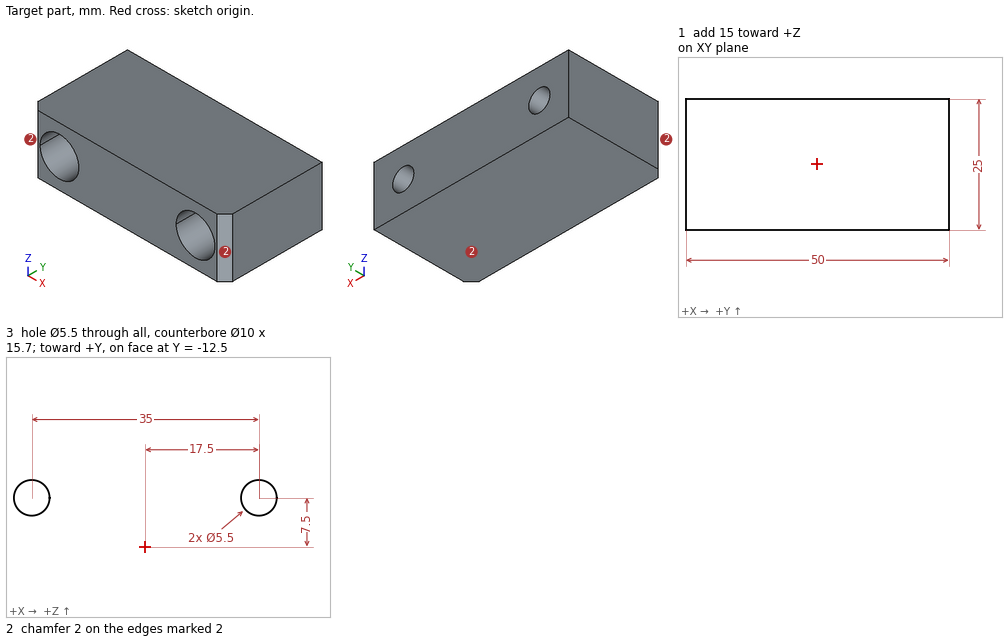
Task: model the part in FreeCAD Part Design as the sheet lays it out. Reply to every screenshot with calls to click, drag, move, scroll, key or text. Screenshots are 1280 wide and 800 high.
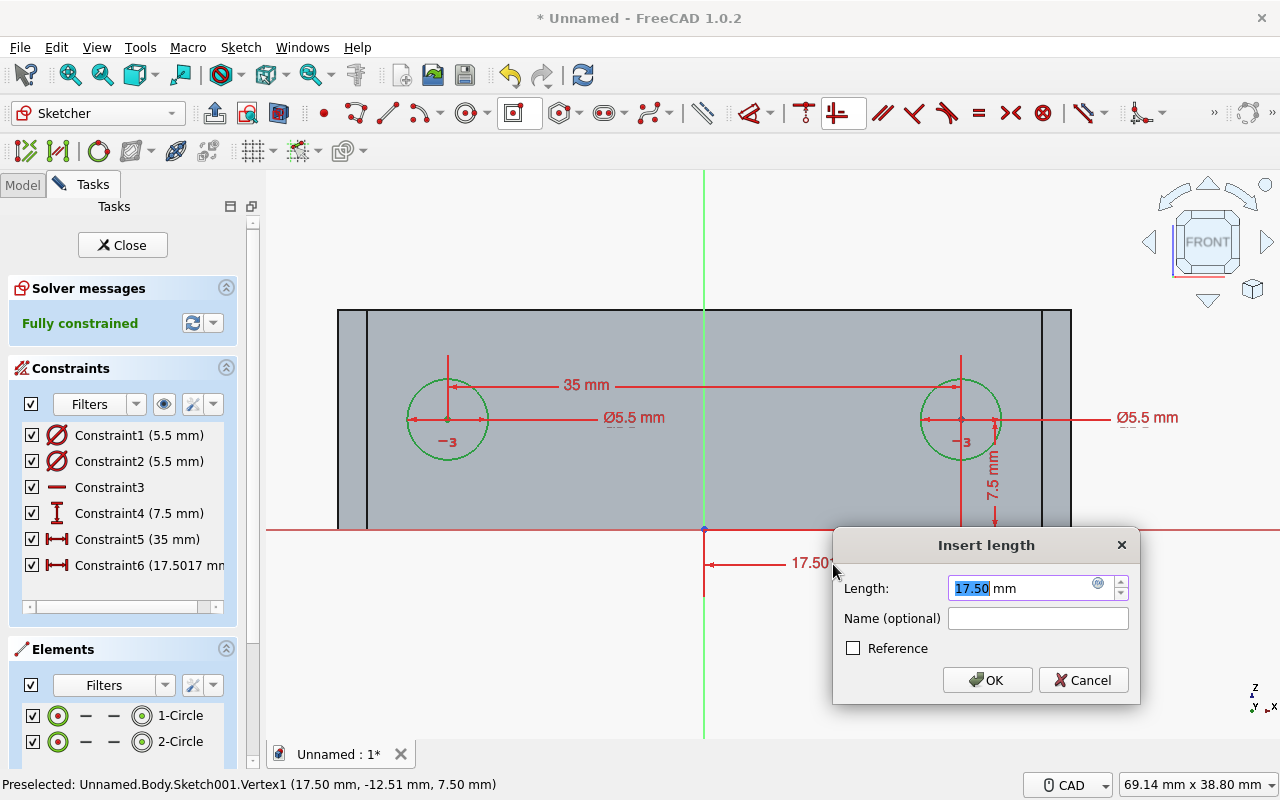
text(17.5)
key(Return)
key(Escape)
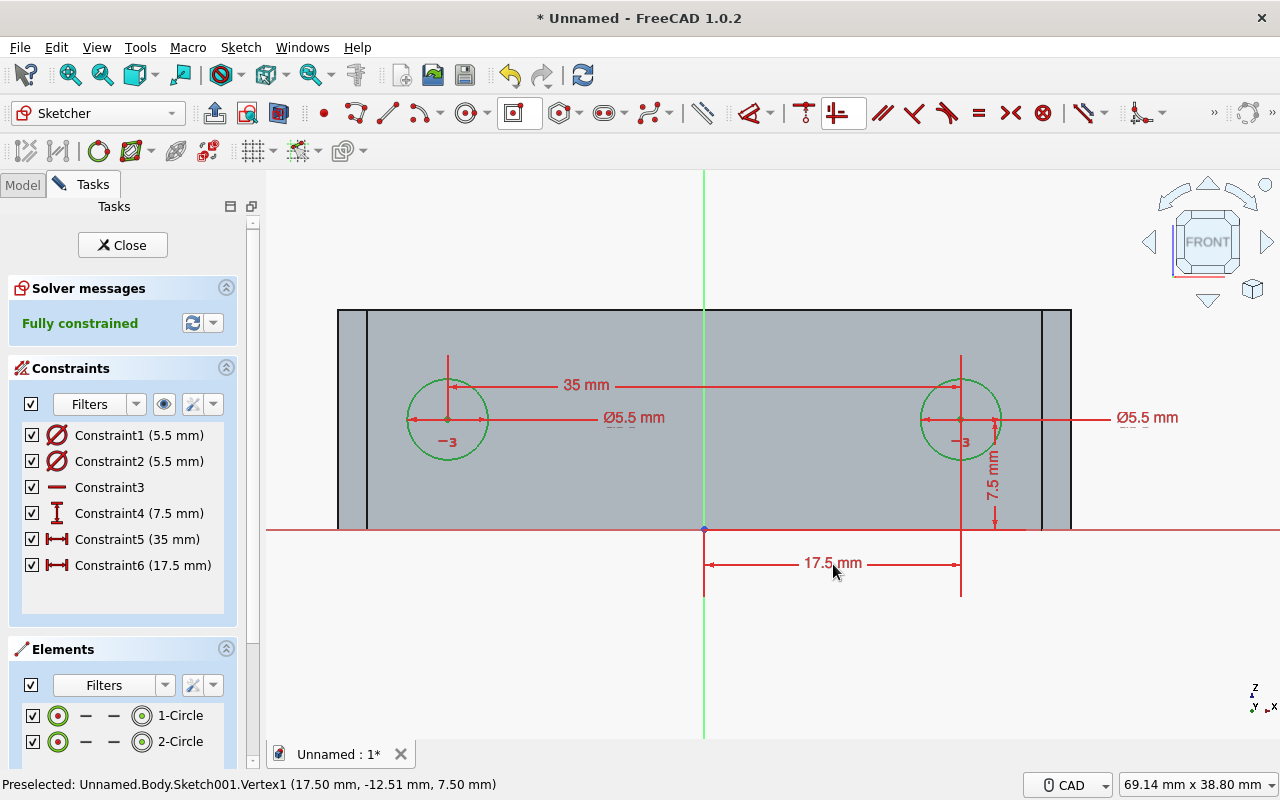
click(123, 245)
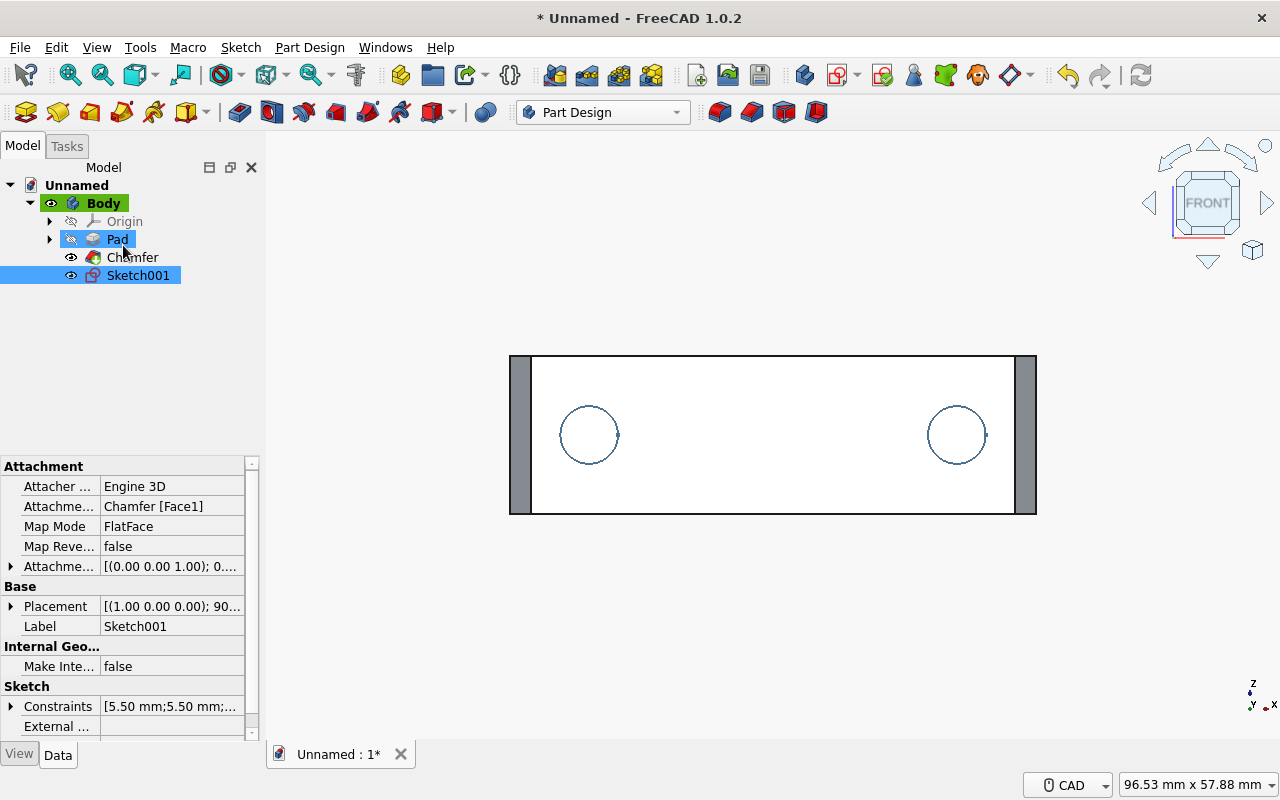
click(272, 112)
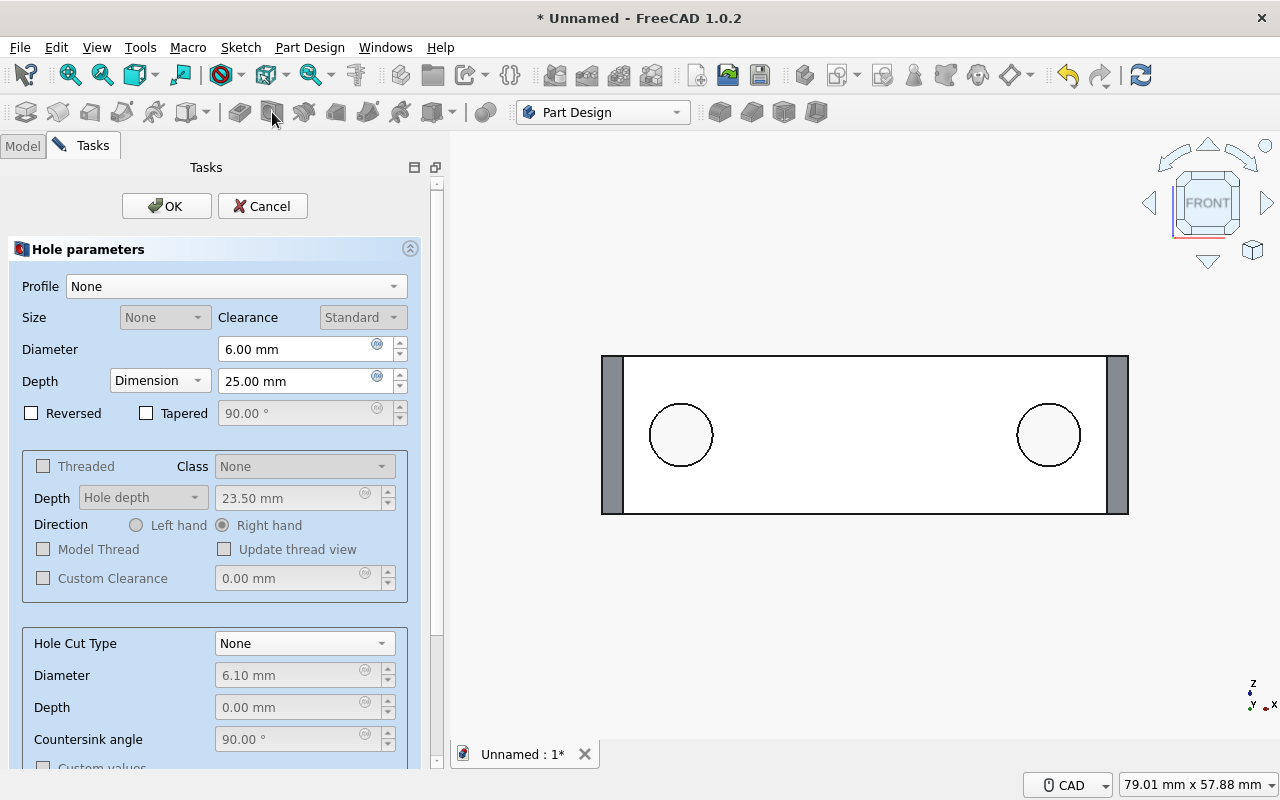
triple_click(305, 349)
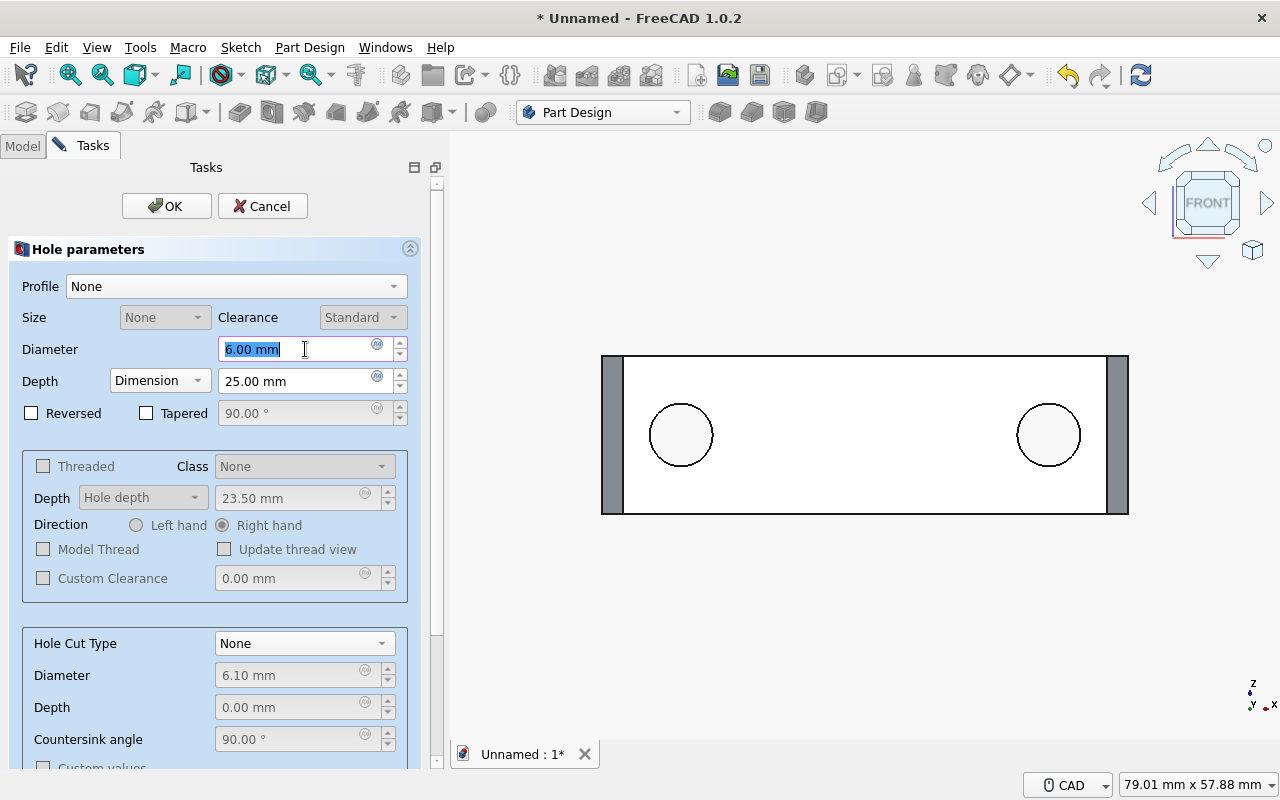
text(5.5)
key(Tab)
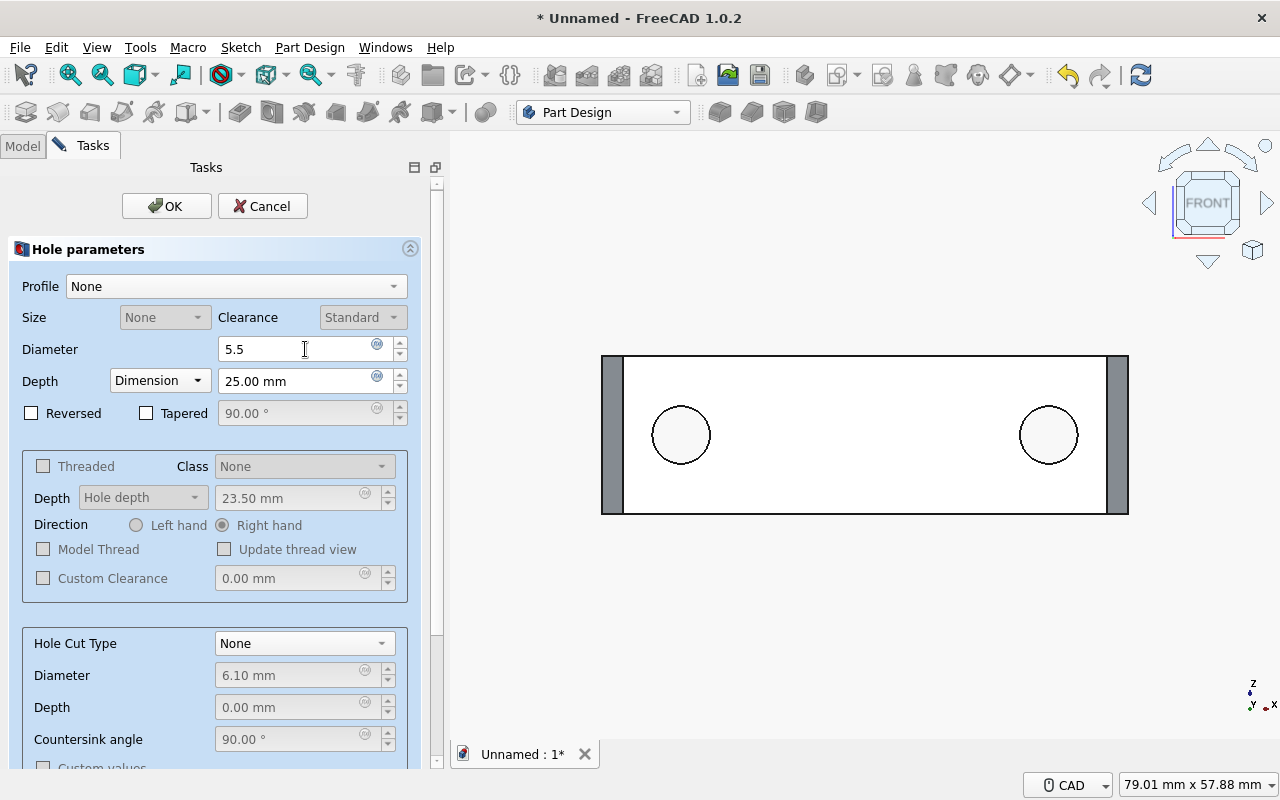
click(161, 380)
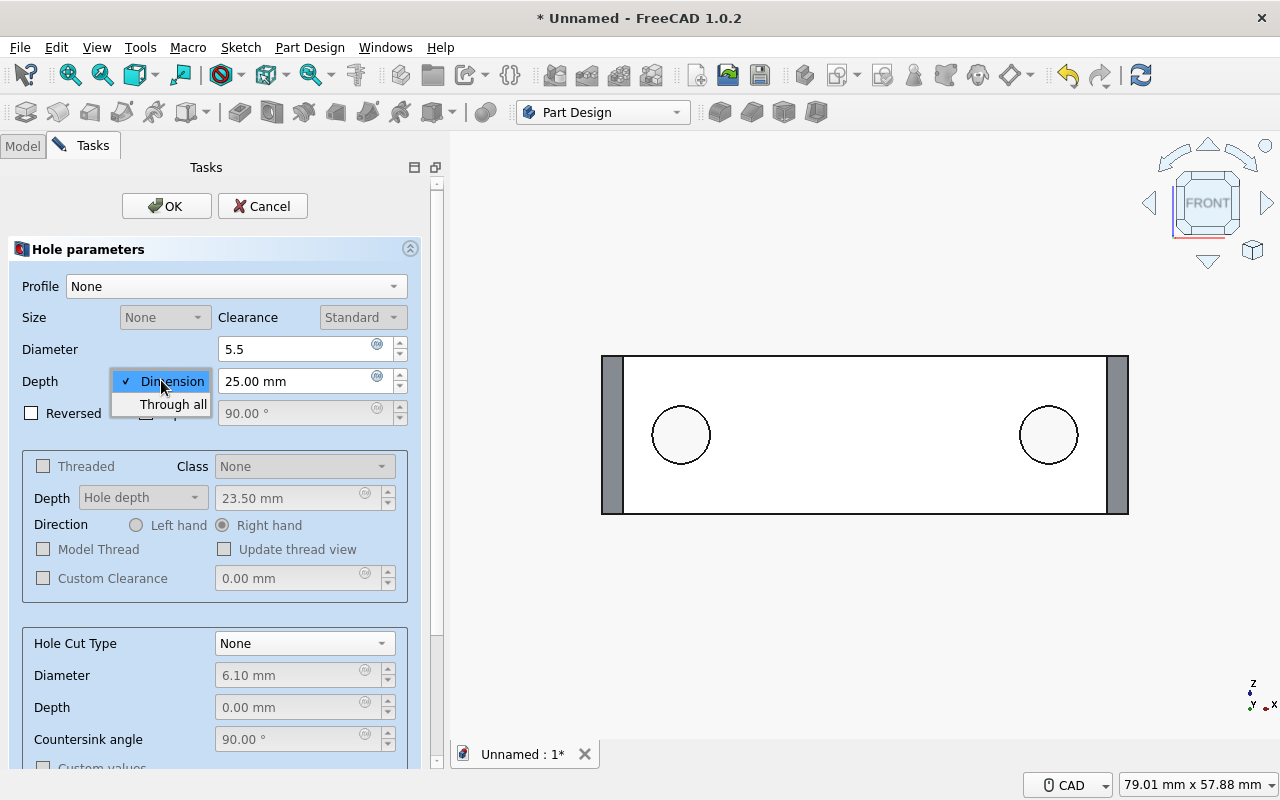
click(160, 404)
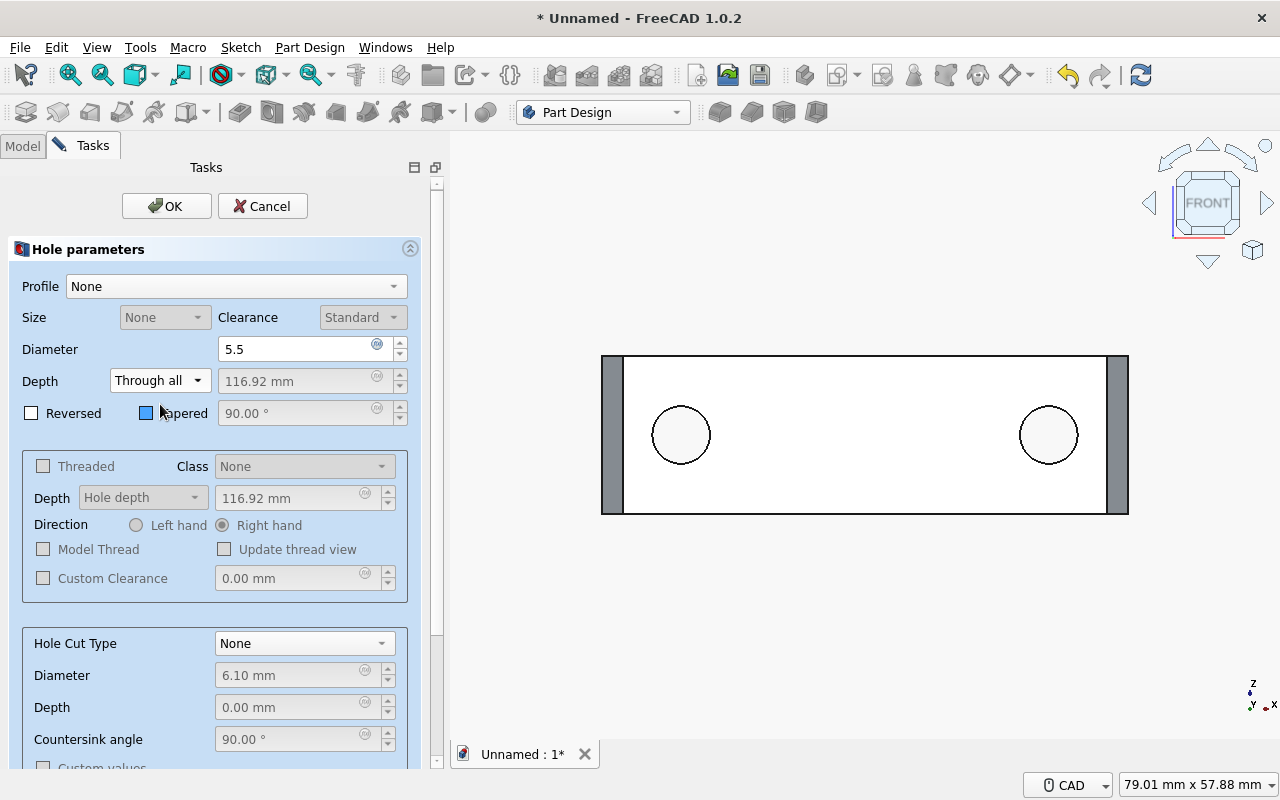
click(306, 644)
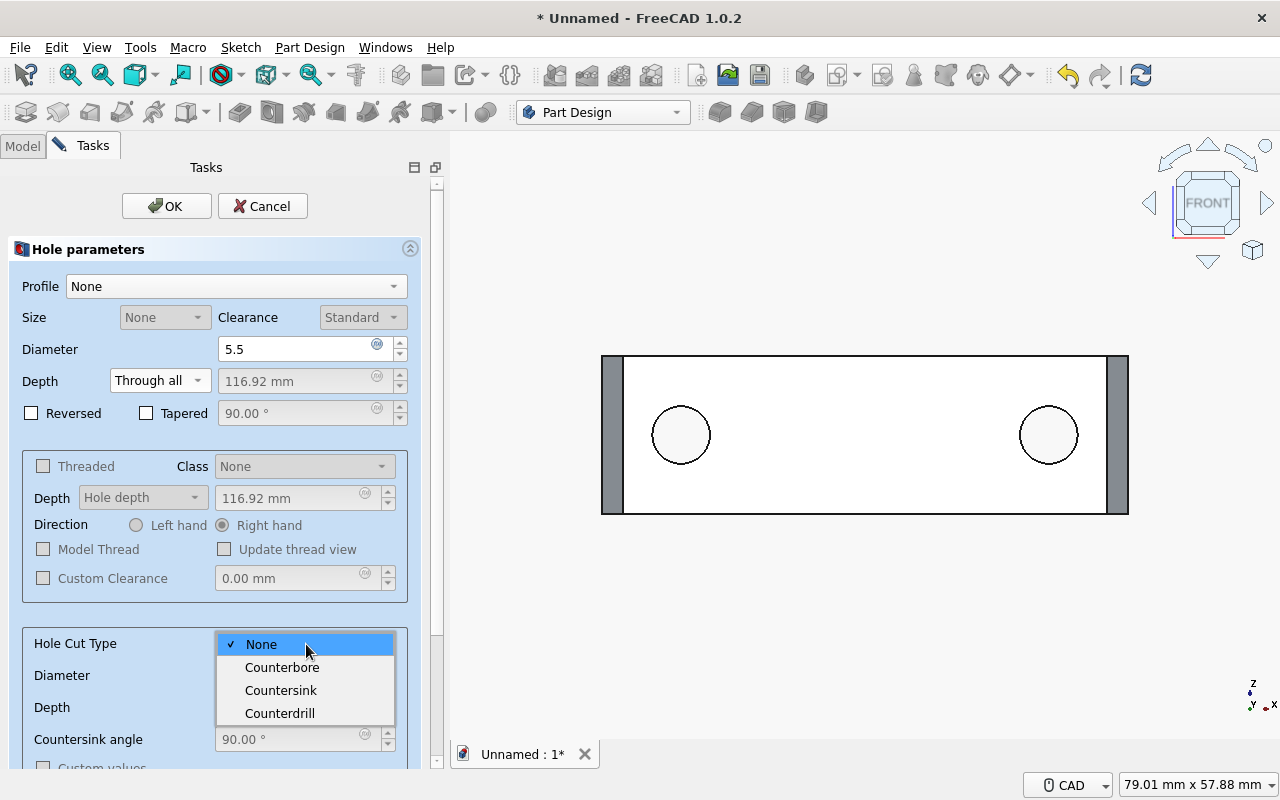
click(304, 668)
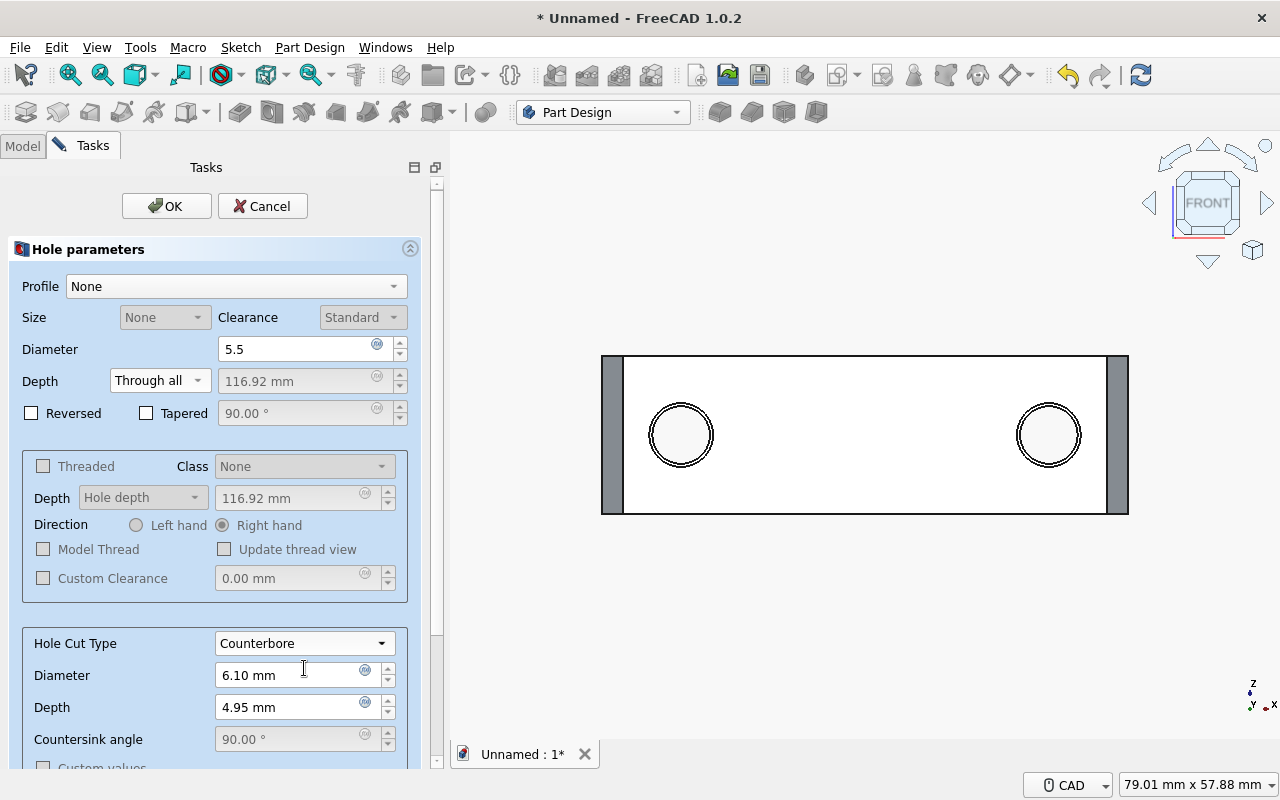
triple_click(298, 675)